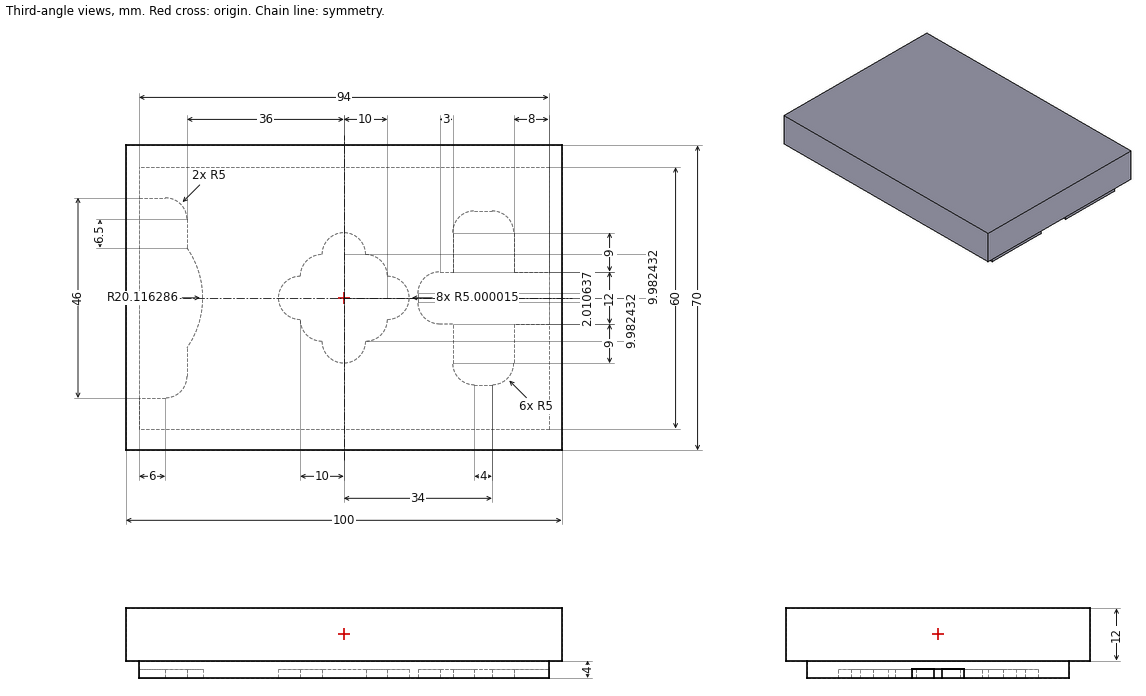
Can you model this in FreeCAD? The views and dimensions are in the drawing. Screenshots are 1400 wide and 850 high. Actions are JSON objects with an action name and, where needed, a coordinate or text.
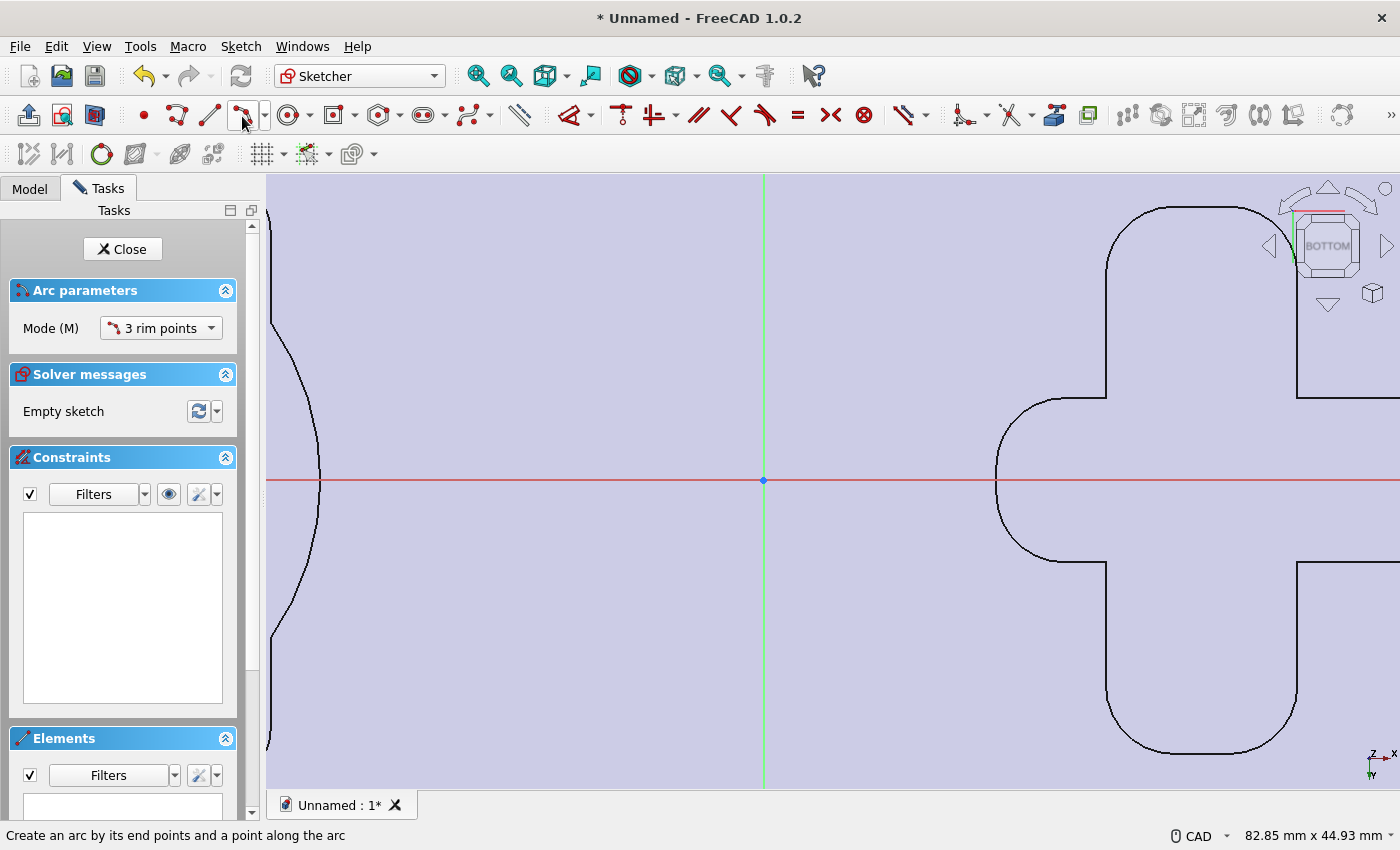
{"action": "left_click", "coordinate": [832, 344]}
{"action": "left_click", "coordinate": [695, 344]}
{"action": "left_click", "coordinate": [785, 279]}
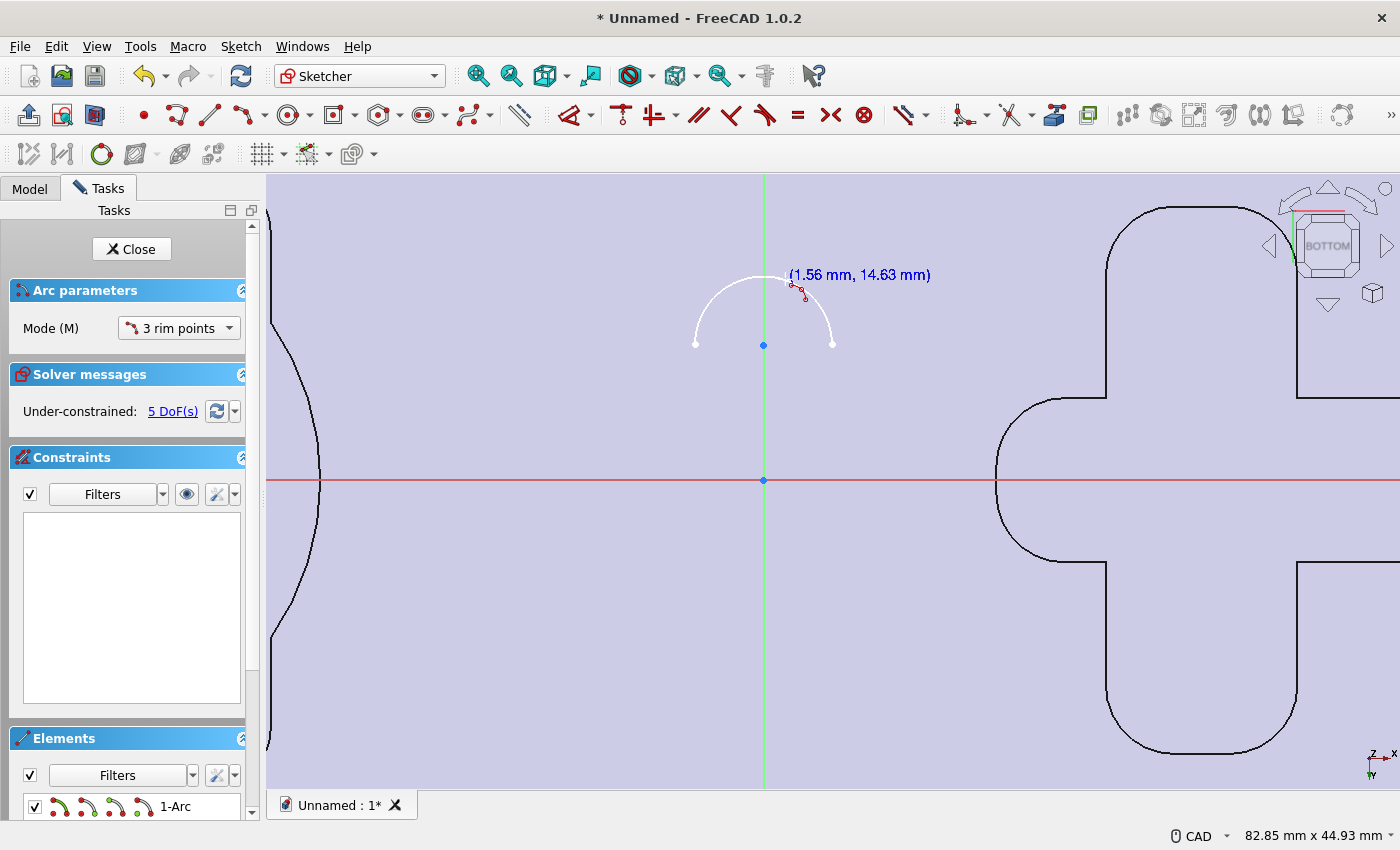
{"action": "left_click", "coordinate": [695, 345]}
{"action": "left_click", "coordinate": [627, 412]}
{"action": "left_click", "coordinate": [647, 364]}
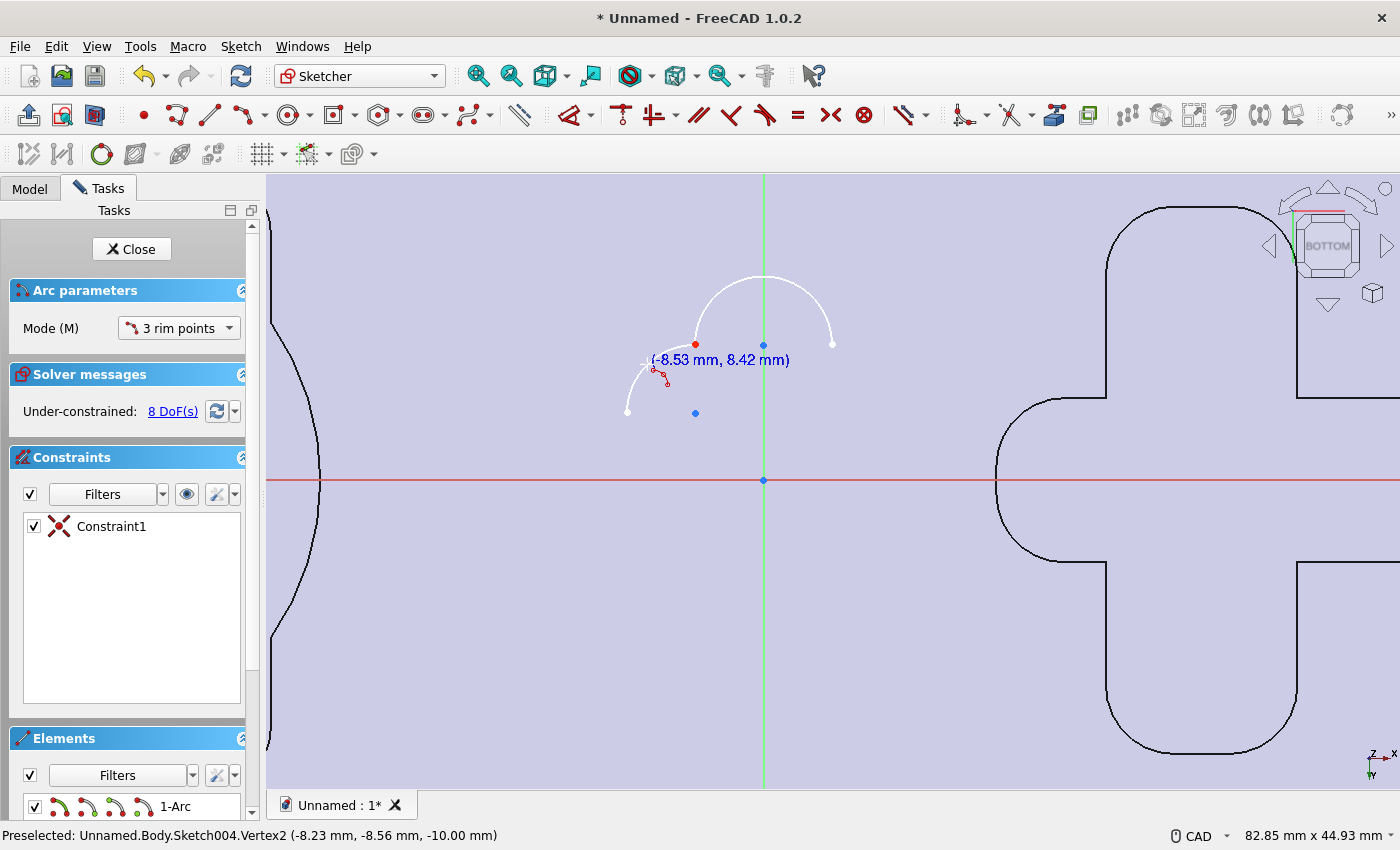
{"action": "left_click", "coordinate": [627, 413]}
{"action": "left_click", "coordinate": [627, 549]}
{"action": "left_click", "coordinate": [562, 459]}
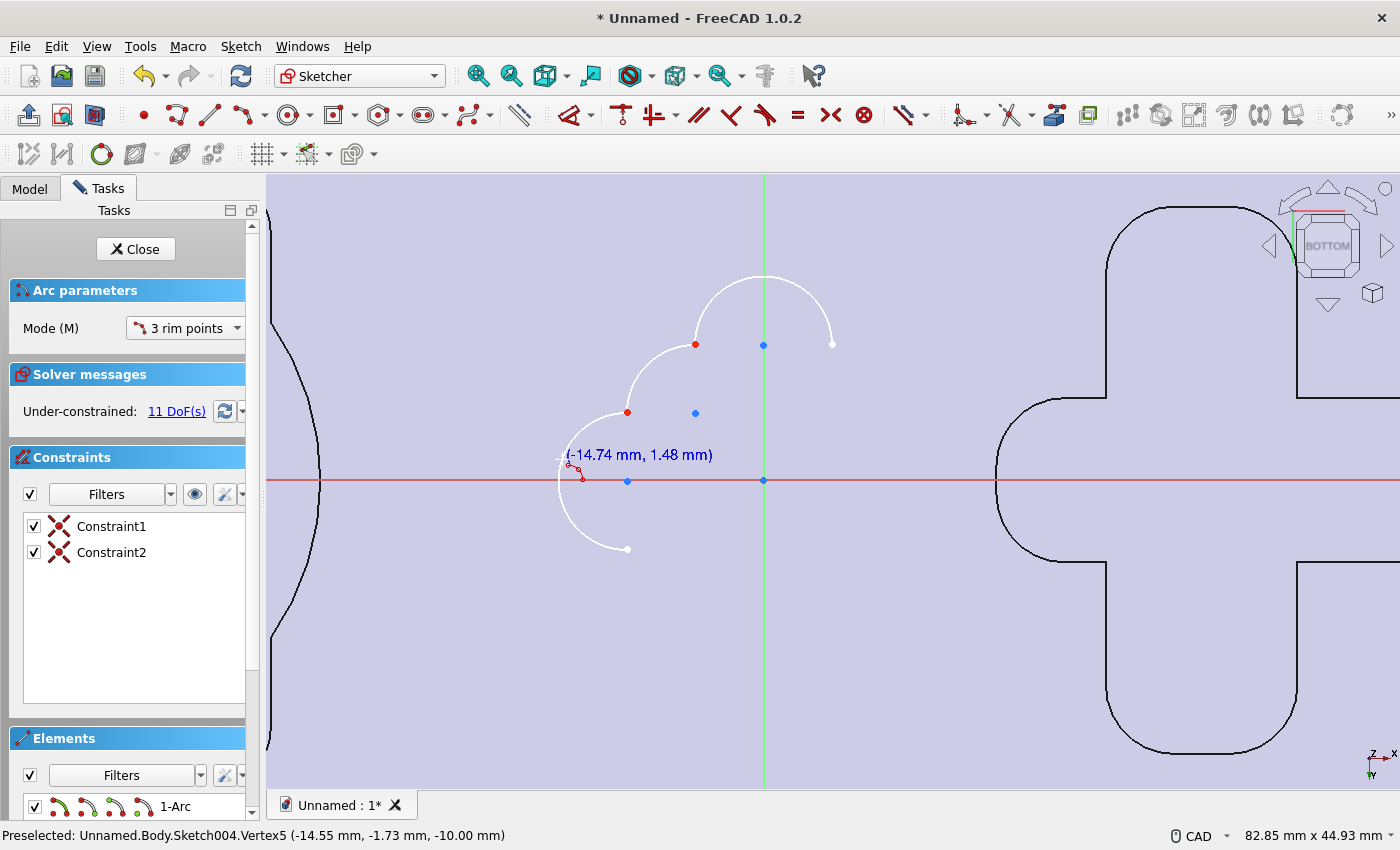
{"action": "left_click", "coordinate": [627, 550]}
{"action": "left_click", "coordinate": [695, 617]}
{"action": "left_click", "coordinate": [647, 597]}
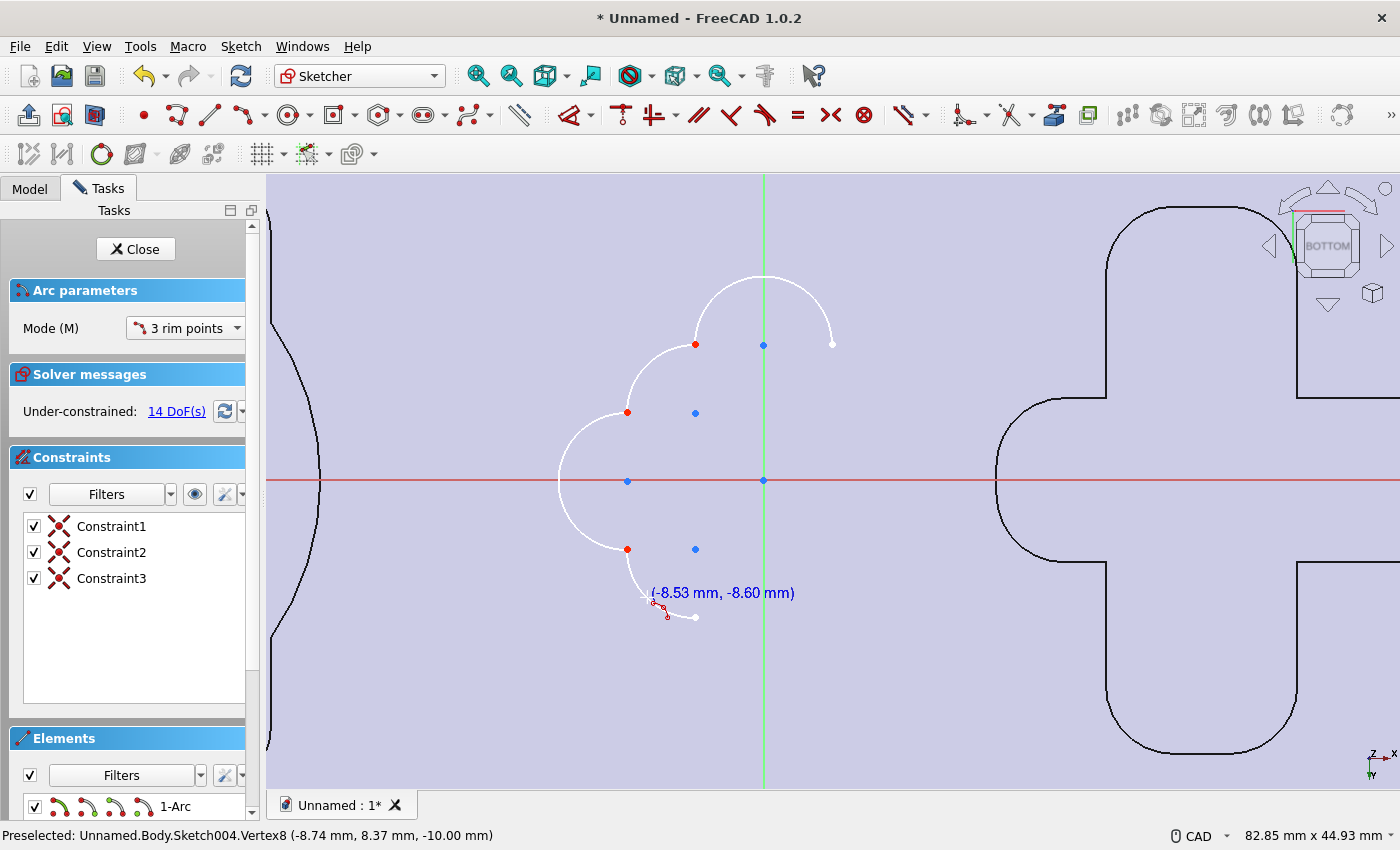
{"action": "left_click", "coordinate": [695, 618]}
{"action": "left_click", "coordinate": [832, 617]}
{"action": "left_click", "coordinate": [743, 682]}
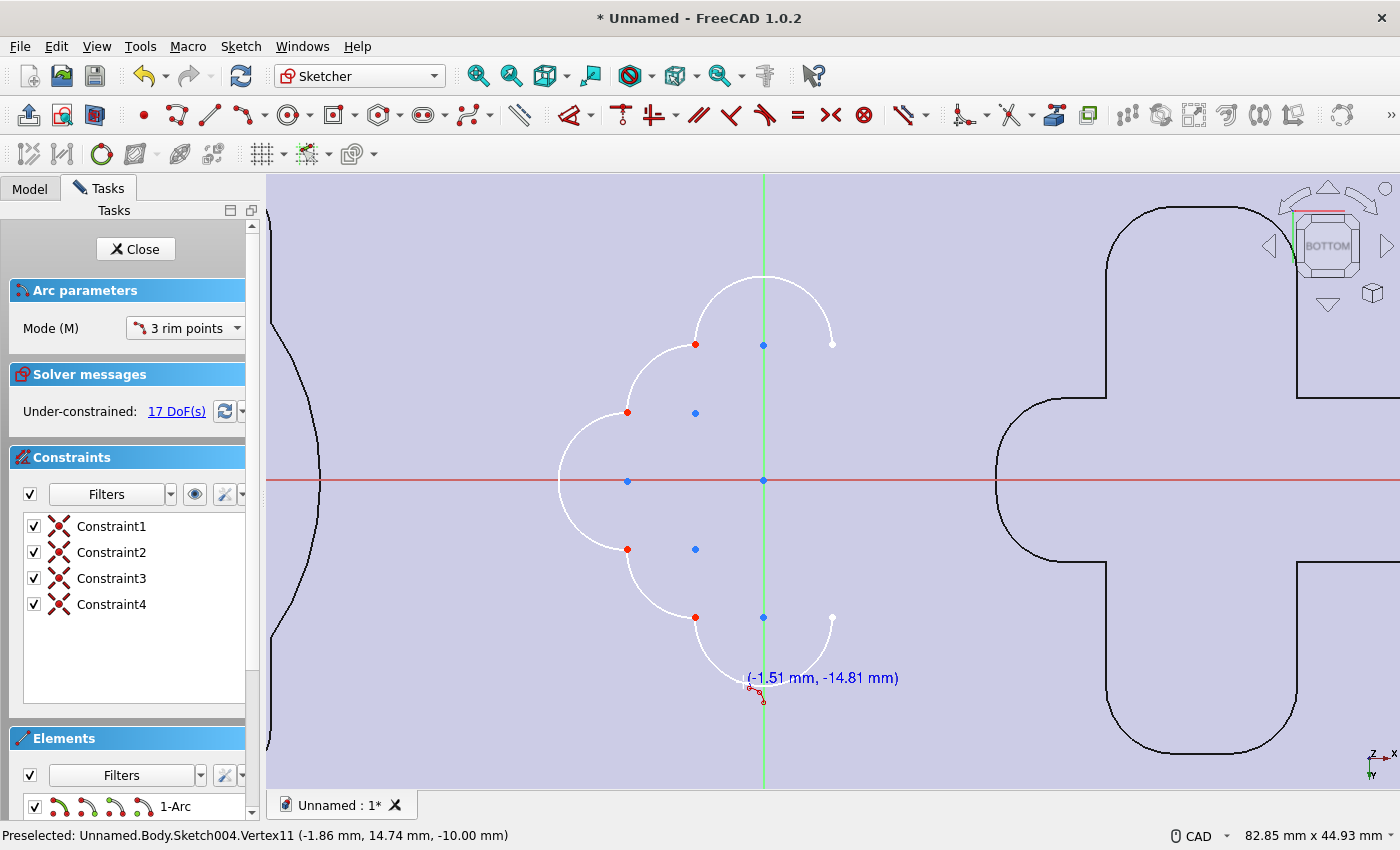
{"action": "left_click", "coordinate": [832, 618]}
{"action": "left_click", "coordinate": [901, 549]}
{"action": "left_click", "coordinate": [880, 597]}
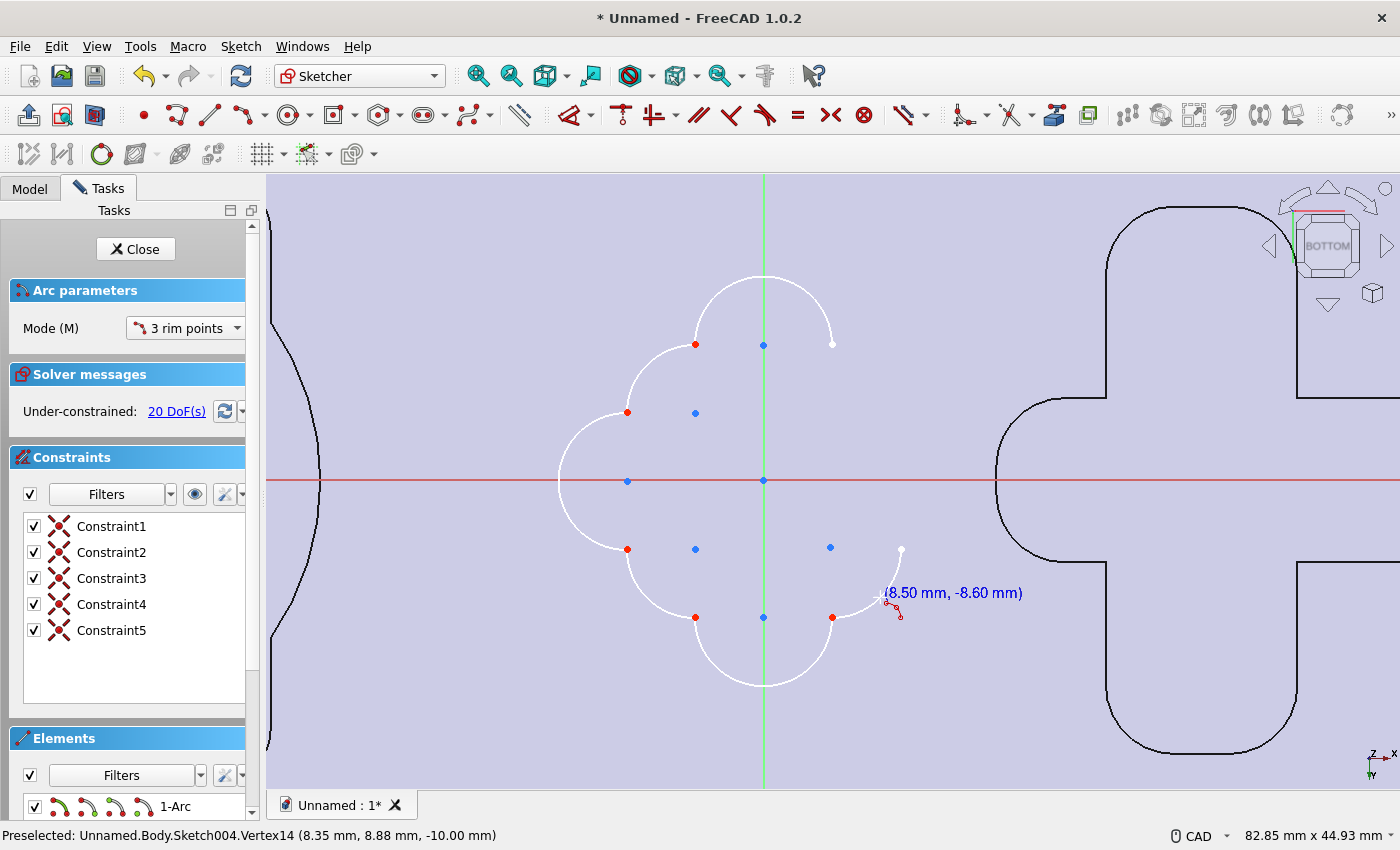
{"action": "left_click", "coordinate": [901, 550]}
{"action": "left_click", "coordinate": [901, 412]}
{"action": "left_click", "coordinate": [966, 501]}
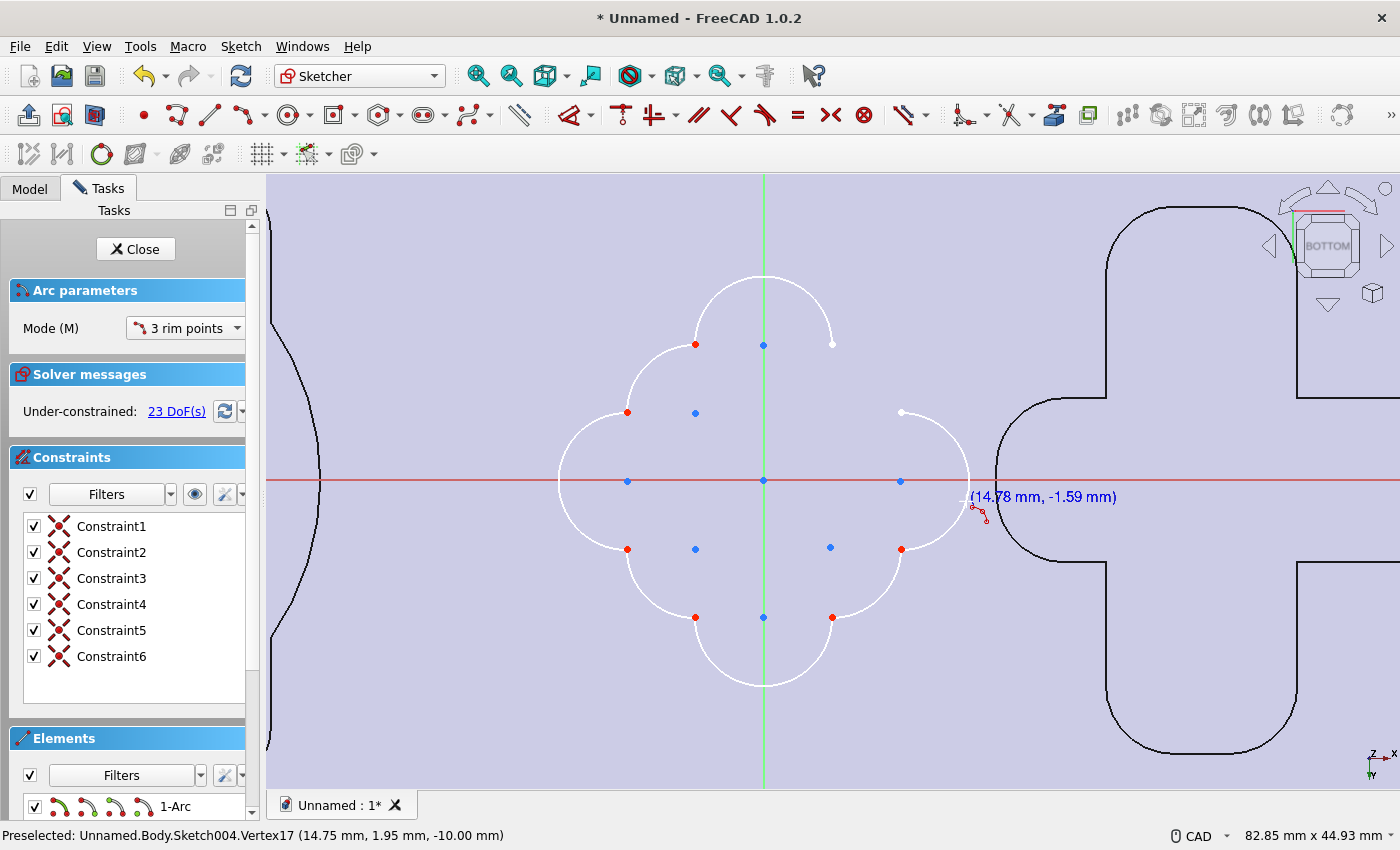
{"action": "left_click", "coordinate": [901, 413]}
{"action": "left_click", "coordinate": [832, 345]}
{"action": "left_click", "coordinate": [880, 364]}
{"action": "key", "text": "Escape"}